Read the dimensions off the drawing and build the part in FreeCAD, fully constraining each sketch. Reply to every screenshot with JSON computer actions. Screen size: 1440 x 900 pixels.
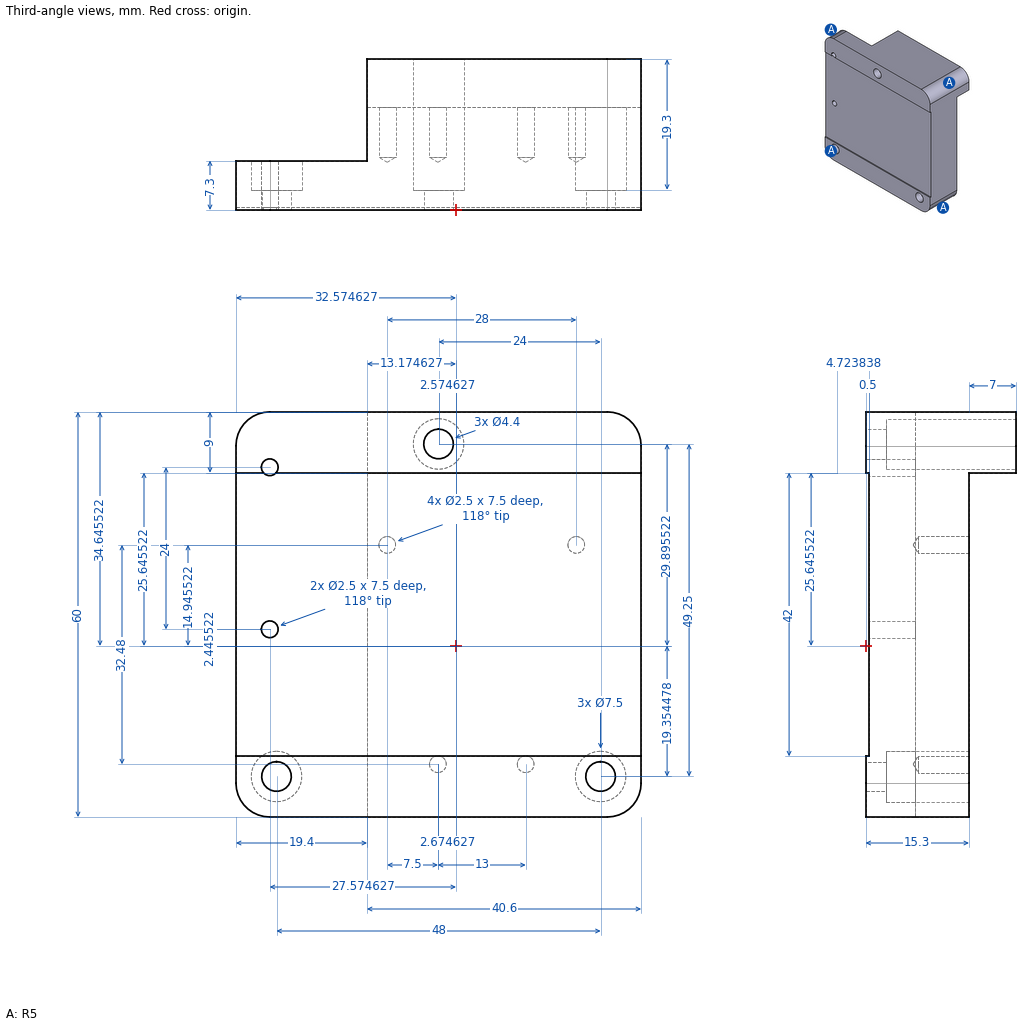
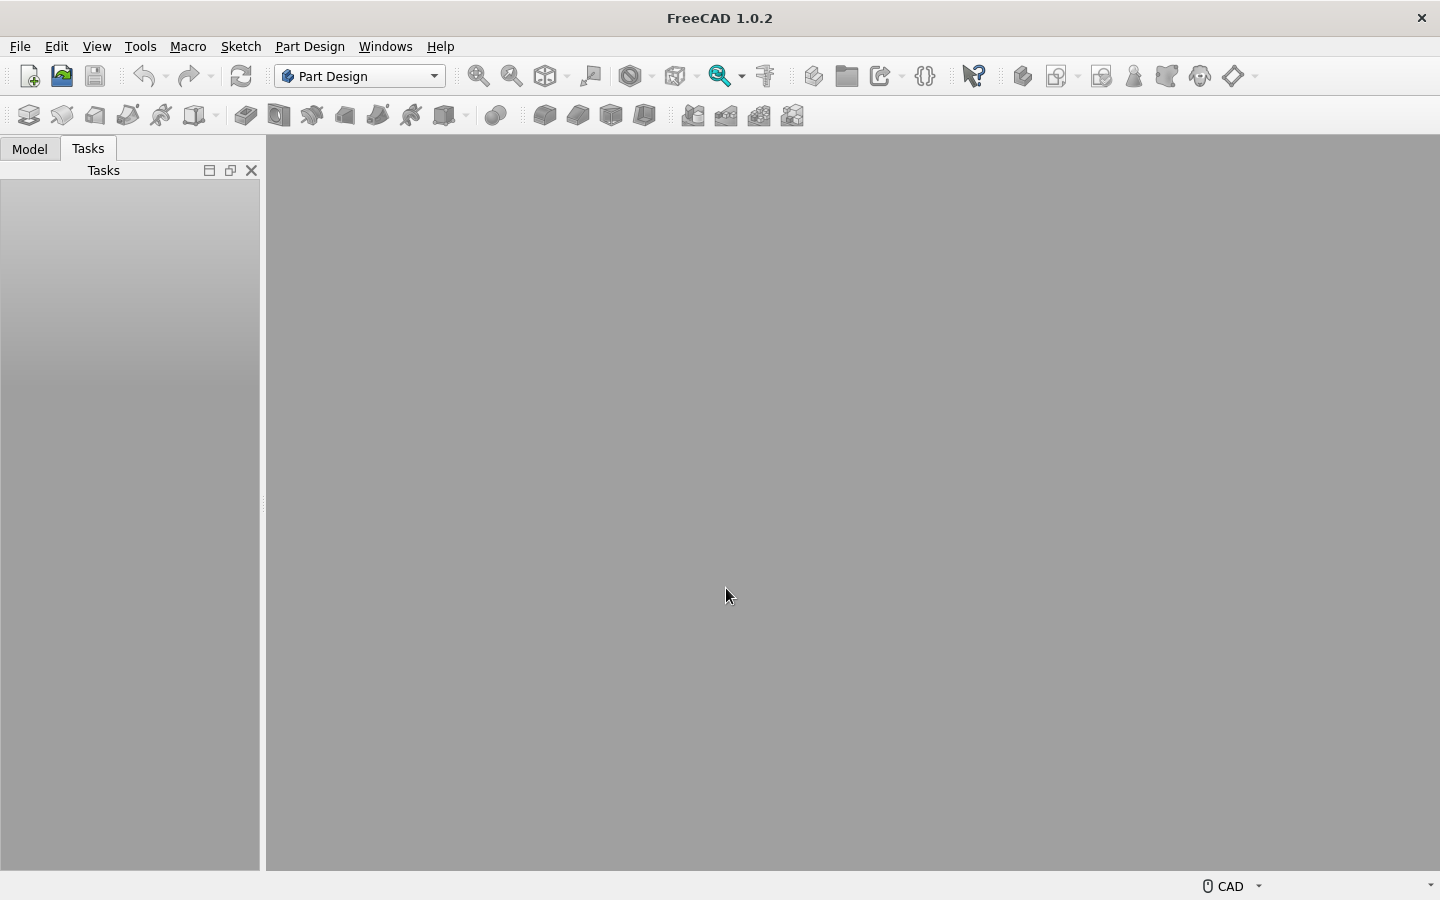
{"action": "left_click", "coordinate": [29, 76]}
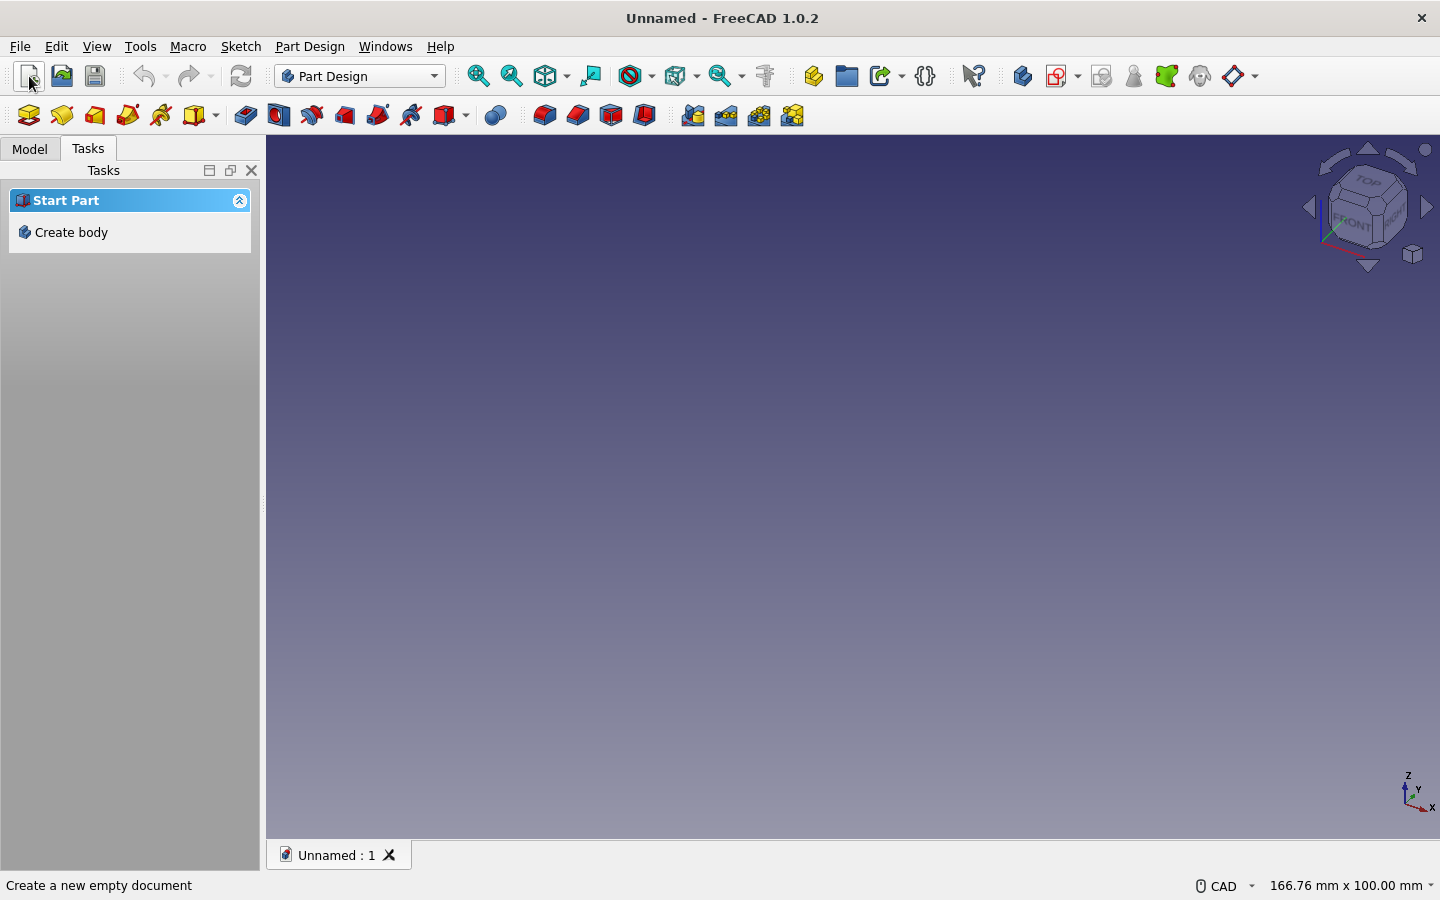
{"action": "left_click", "coordinate": [1056, 76]}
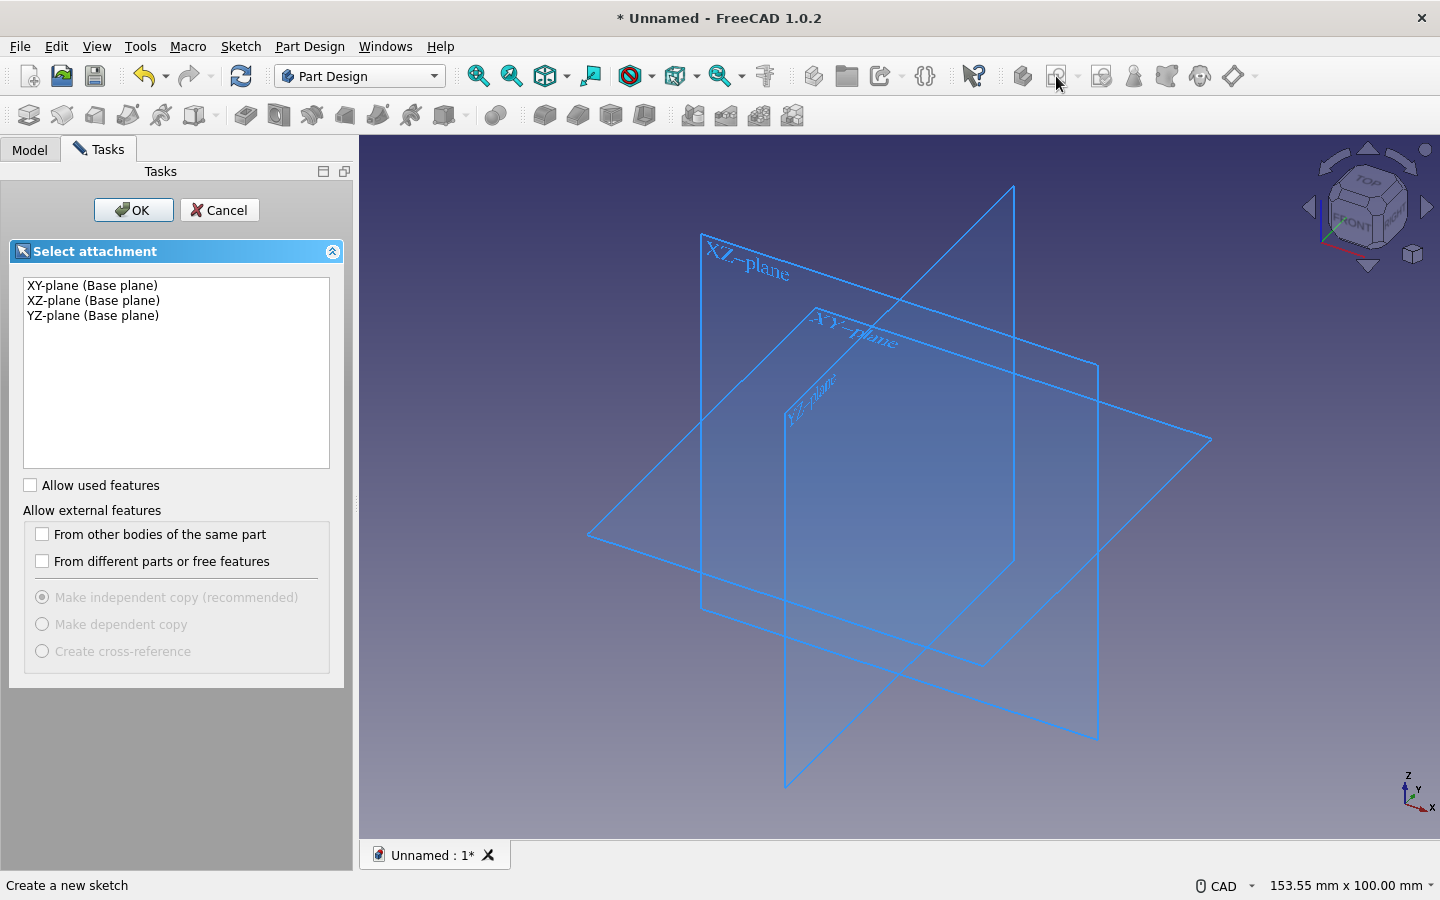
{"action": "left_click", "coordinate": [84, 300]}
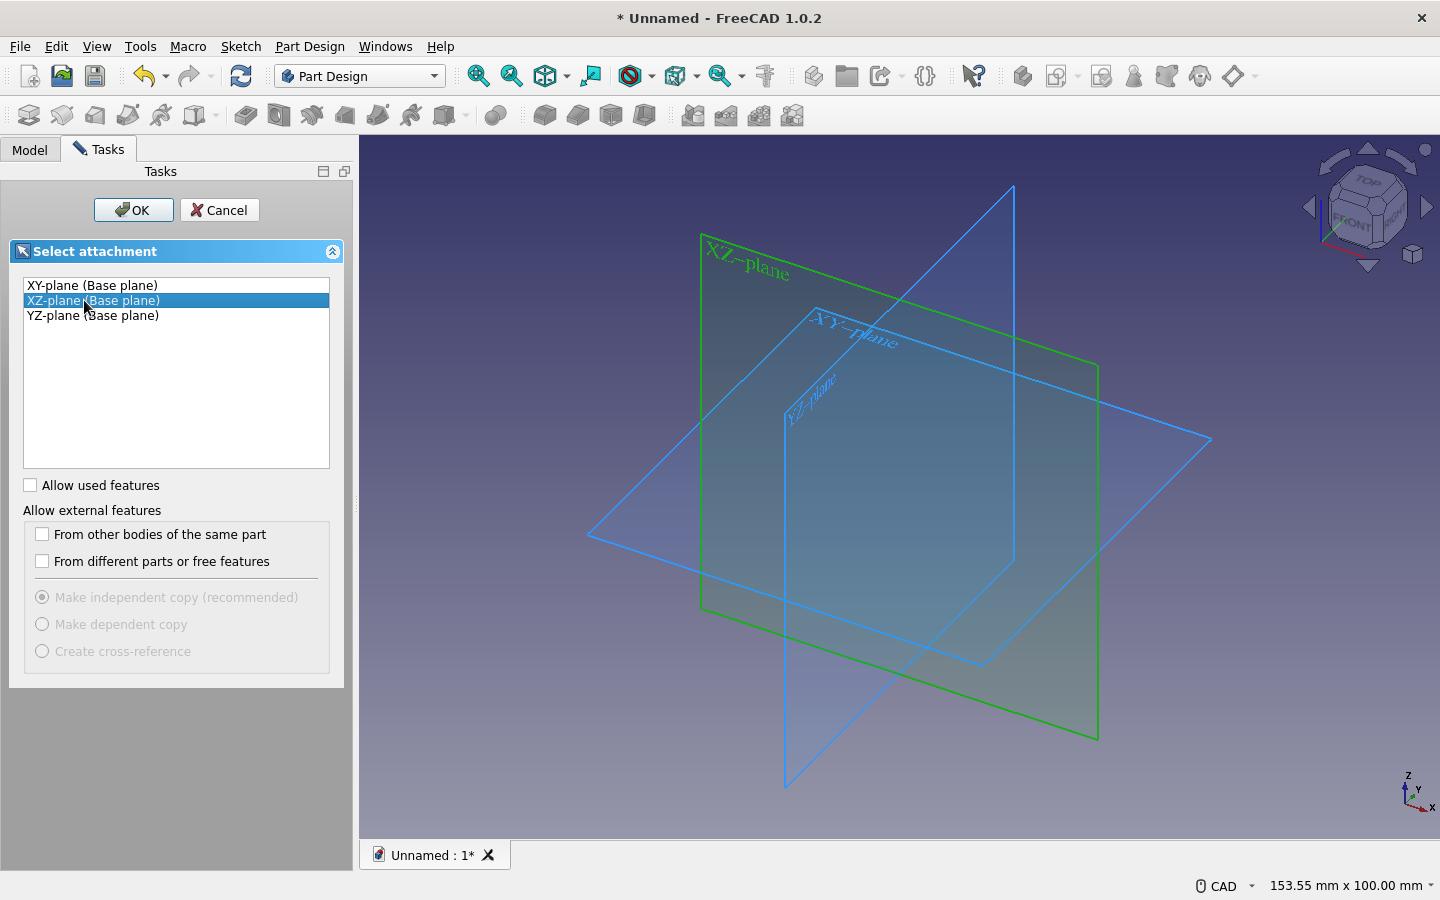
{"action": "left_click", "coordinate": [134, 210]}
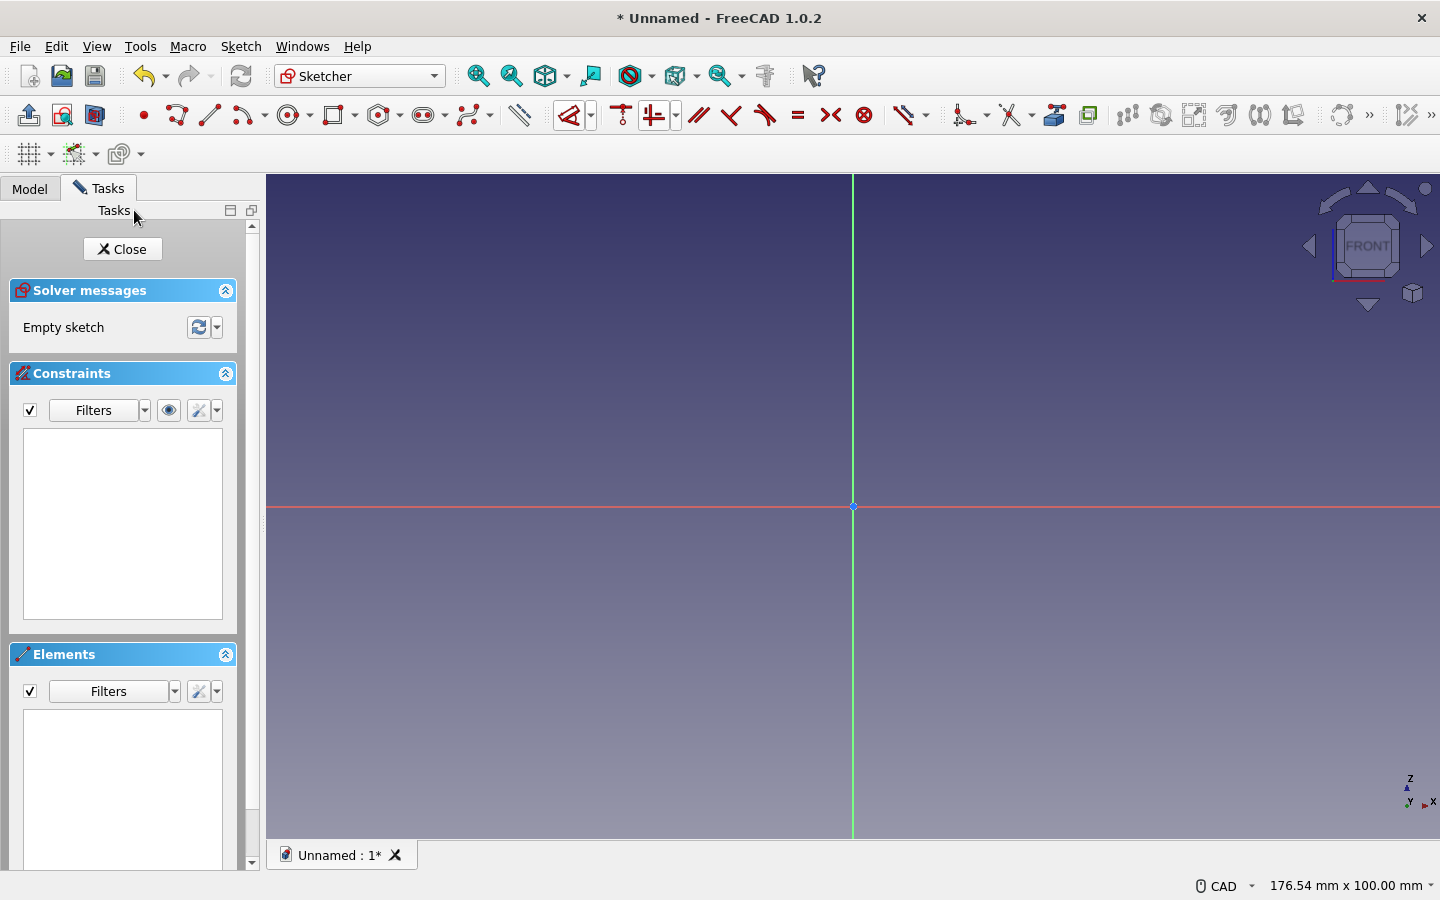
{"action": "key", "text": "g r"}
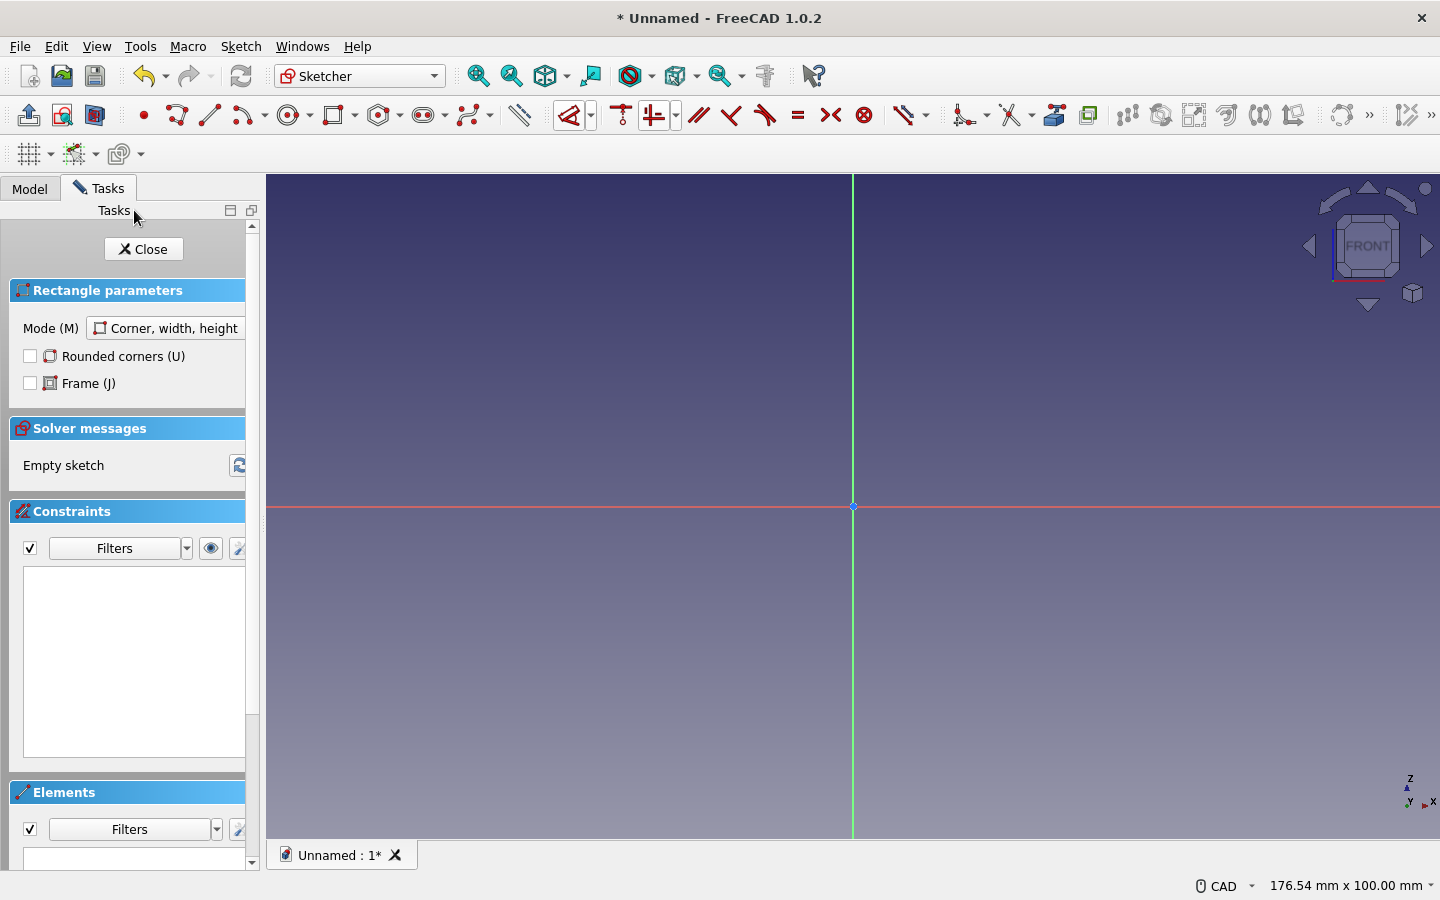
{"action": "left_click", "coordinate": [765, 276]}
{"action": "left_click", "coordinate": [1035, 675]}
{"action": "key", "text": "Escape"}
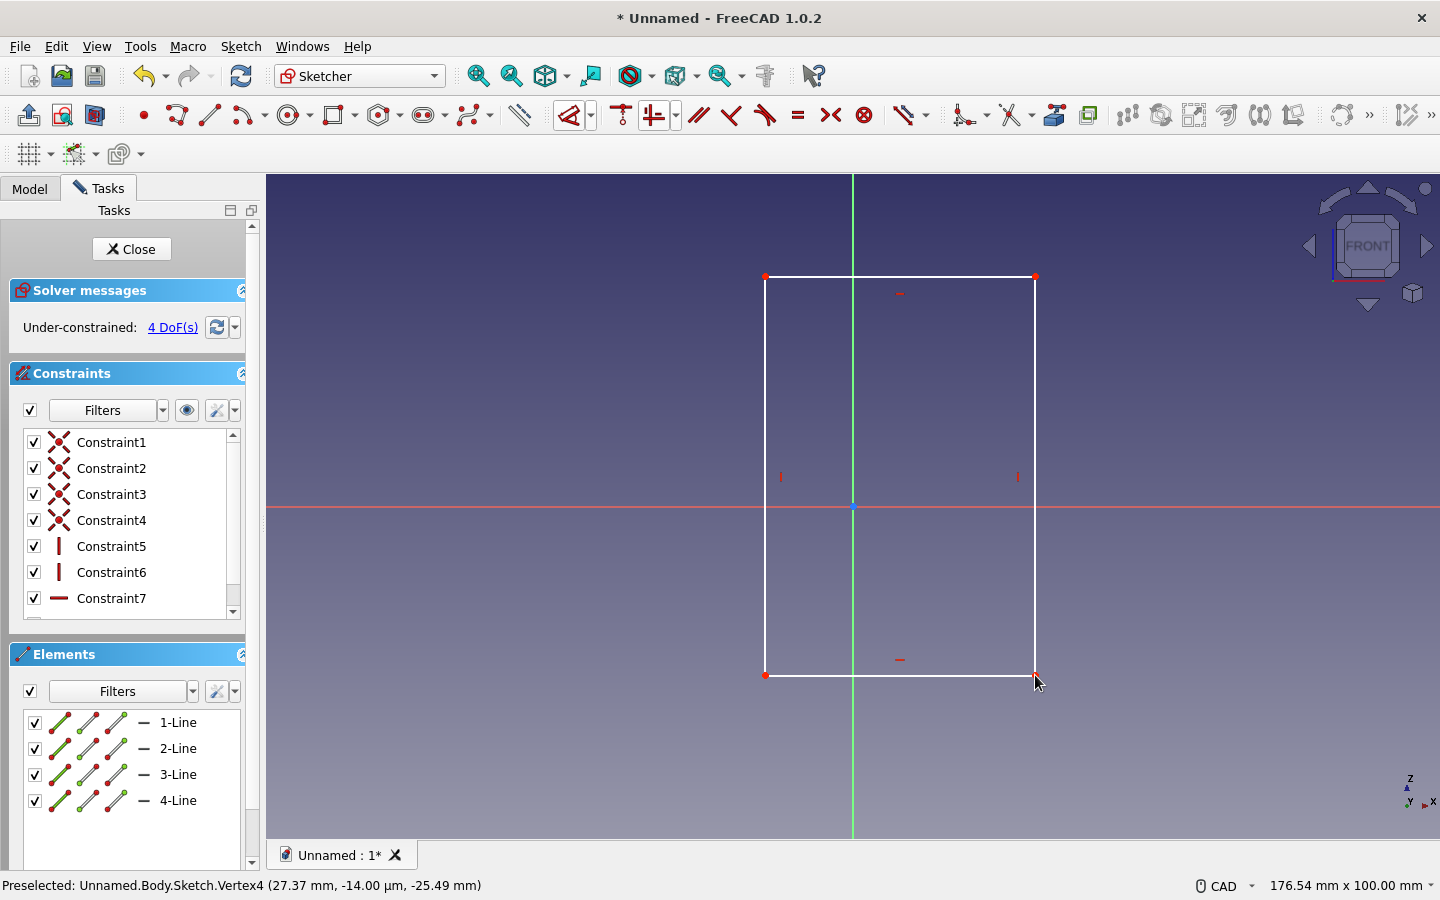
{"action": "key", "text": "d"}